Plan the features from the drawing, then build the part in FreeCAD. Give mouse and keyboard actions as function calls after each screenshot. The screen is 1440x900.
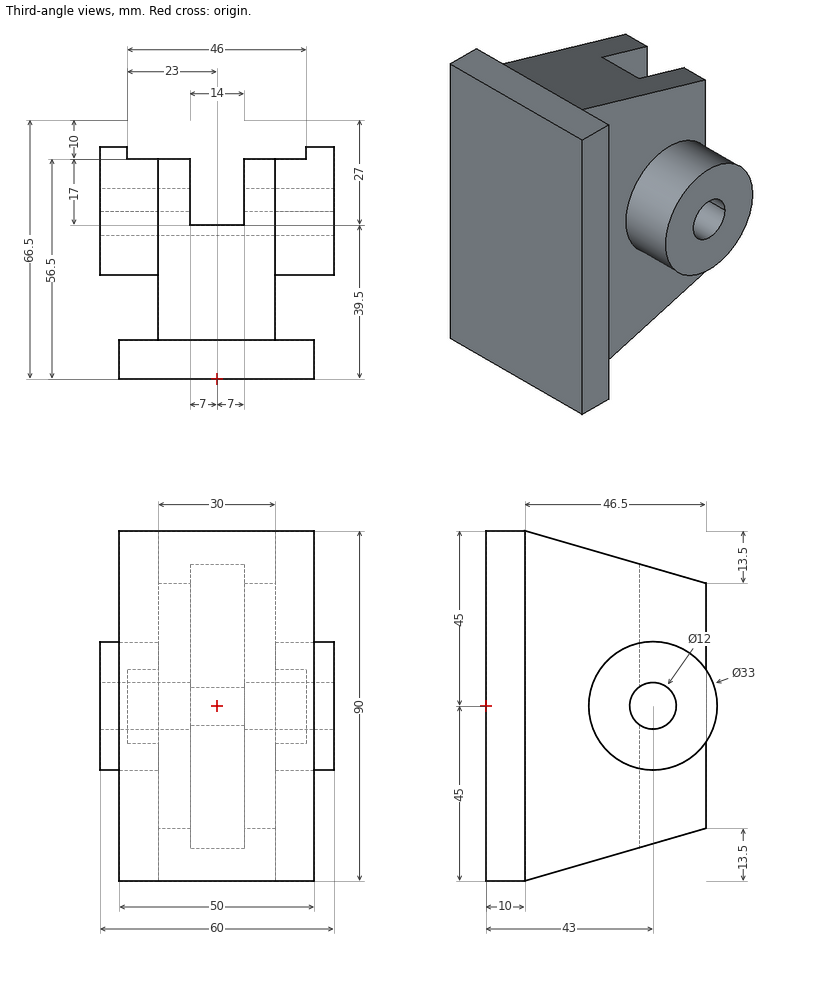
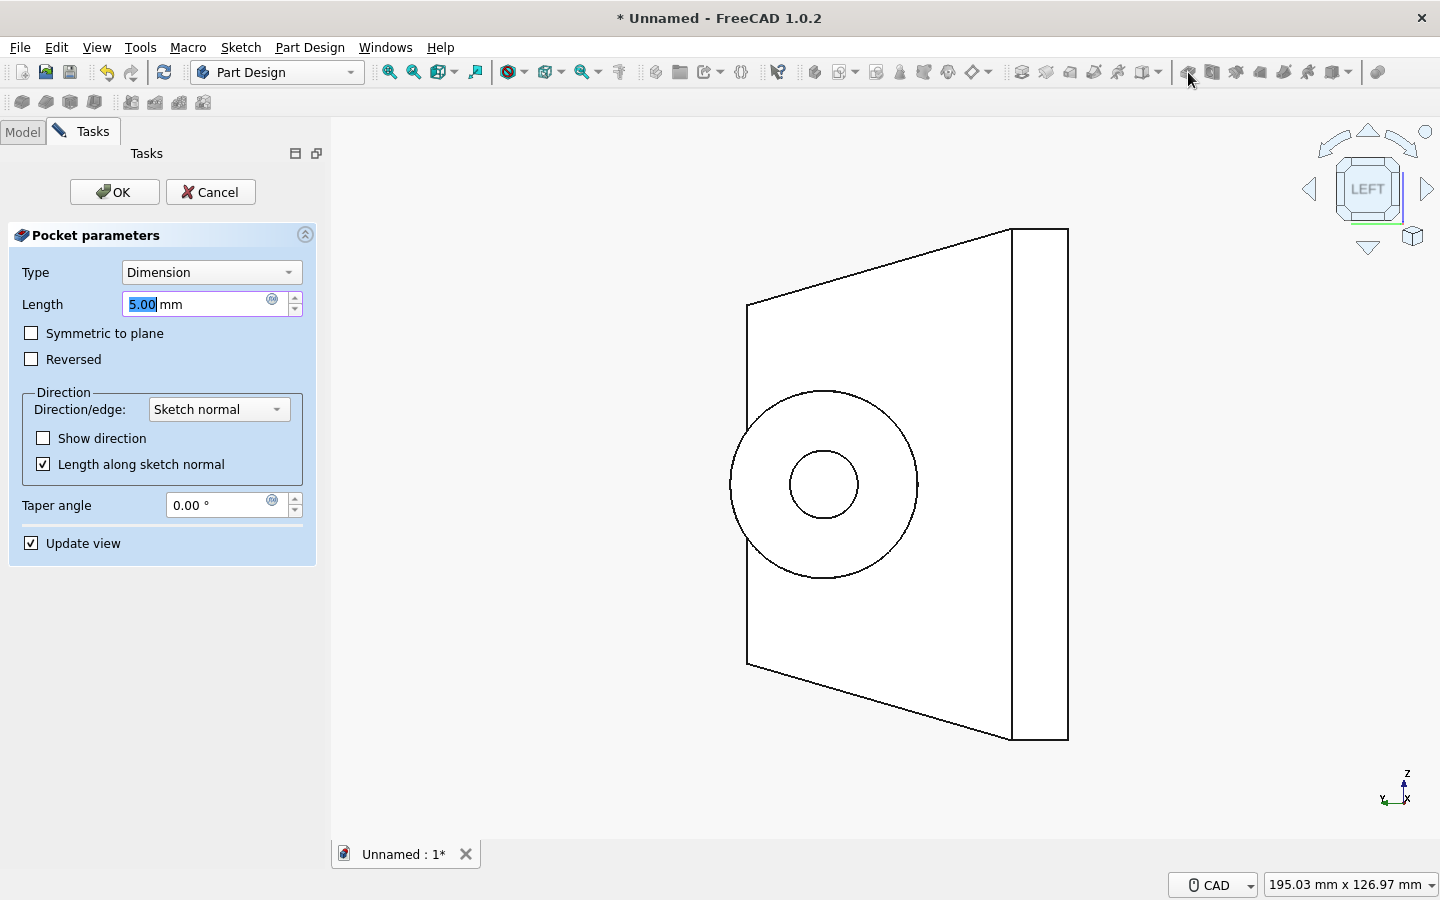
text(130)
key(Tab)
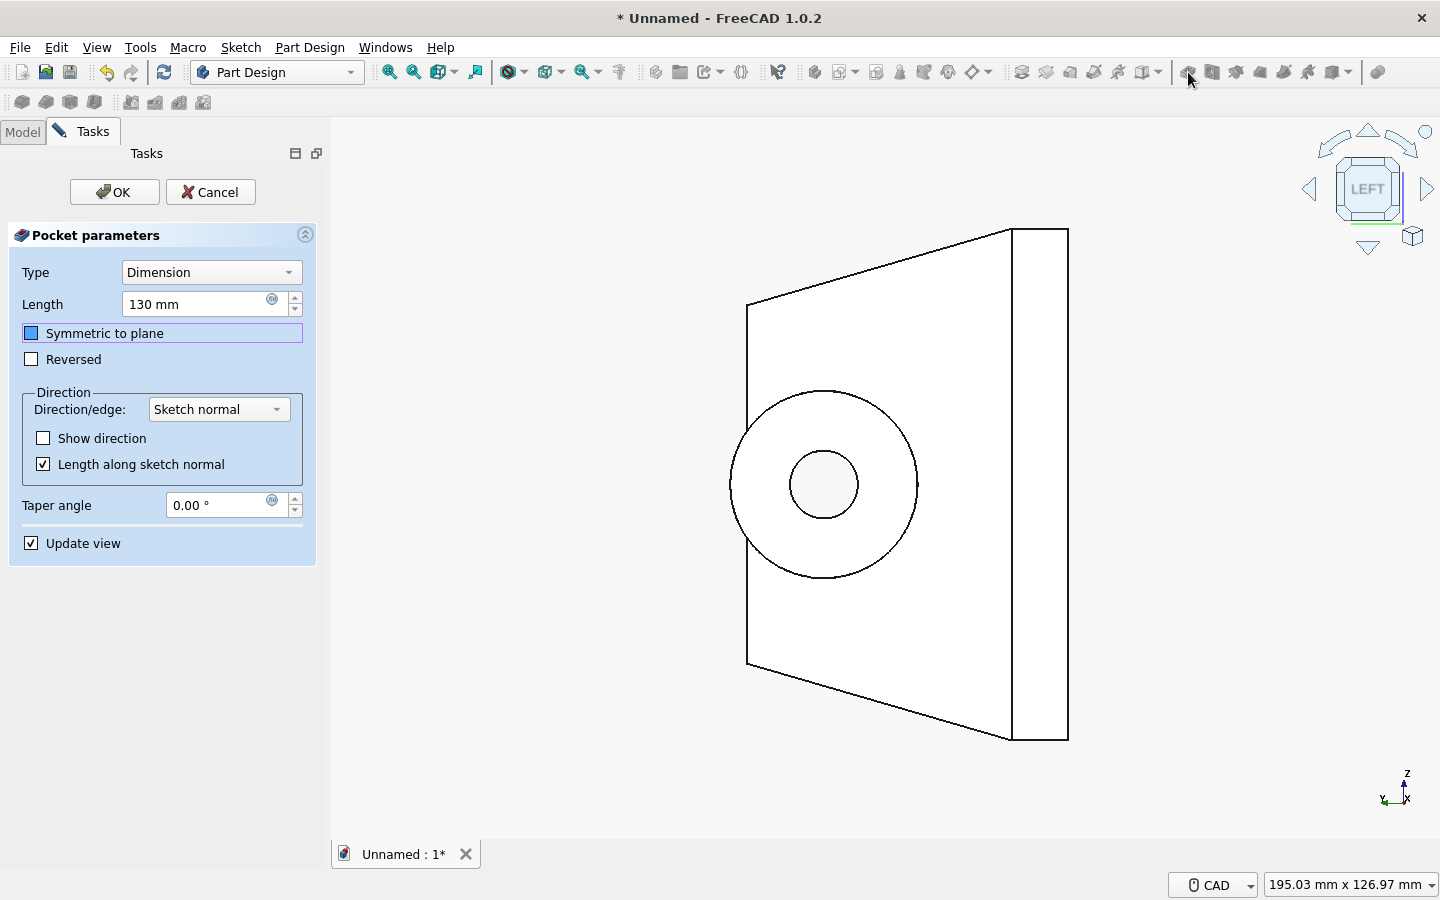
click(30, 333)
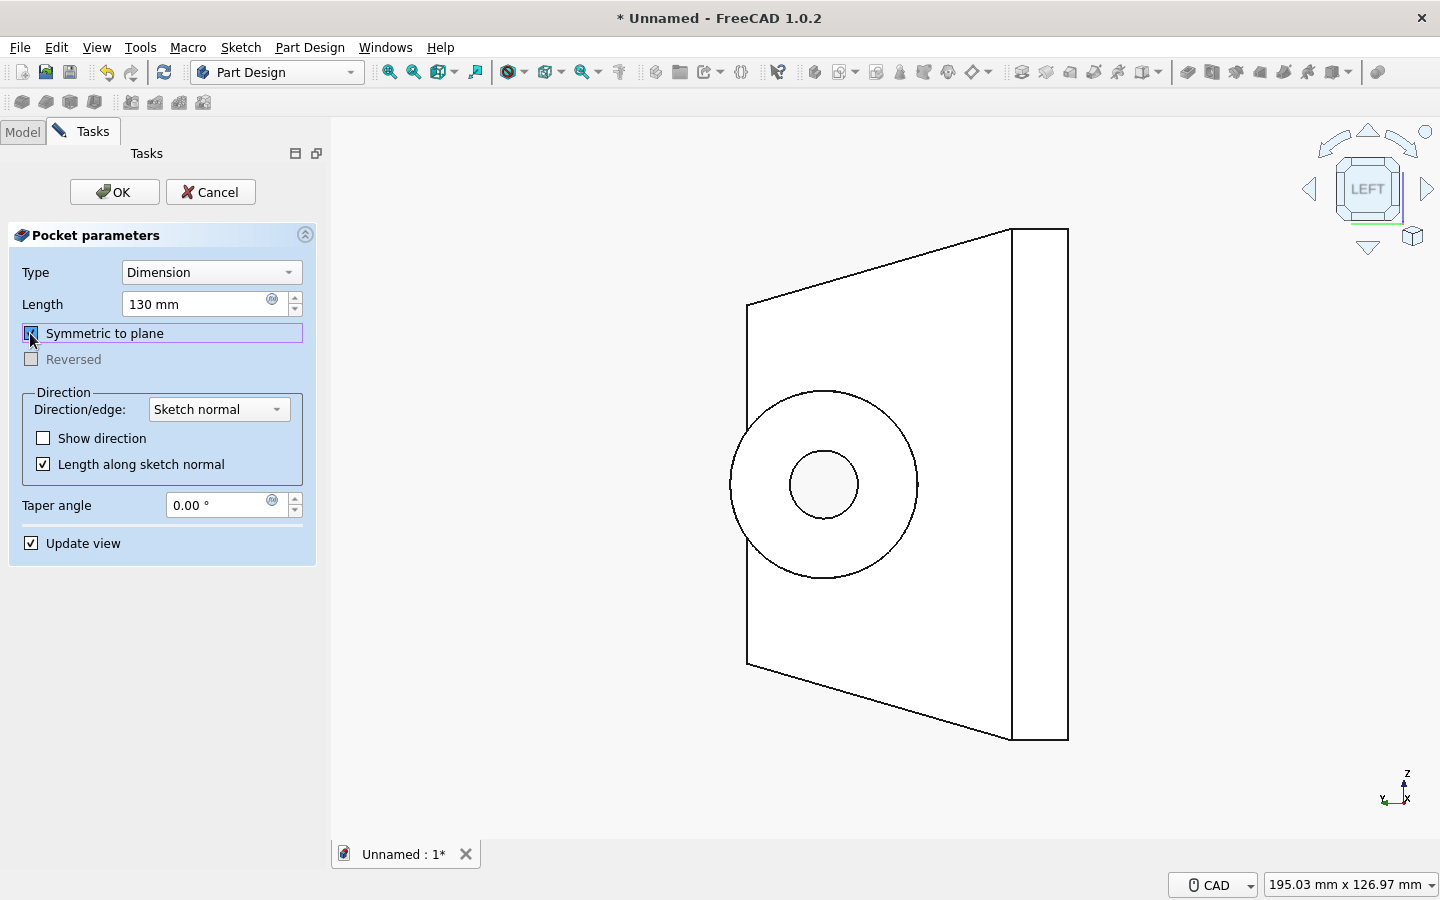
click(115, 192)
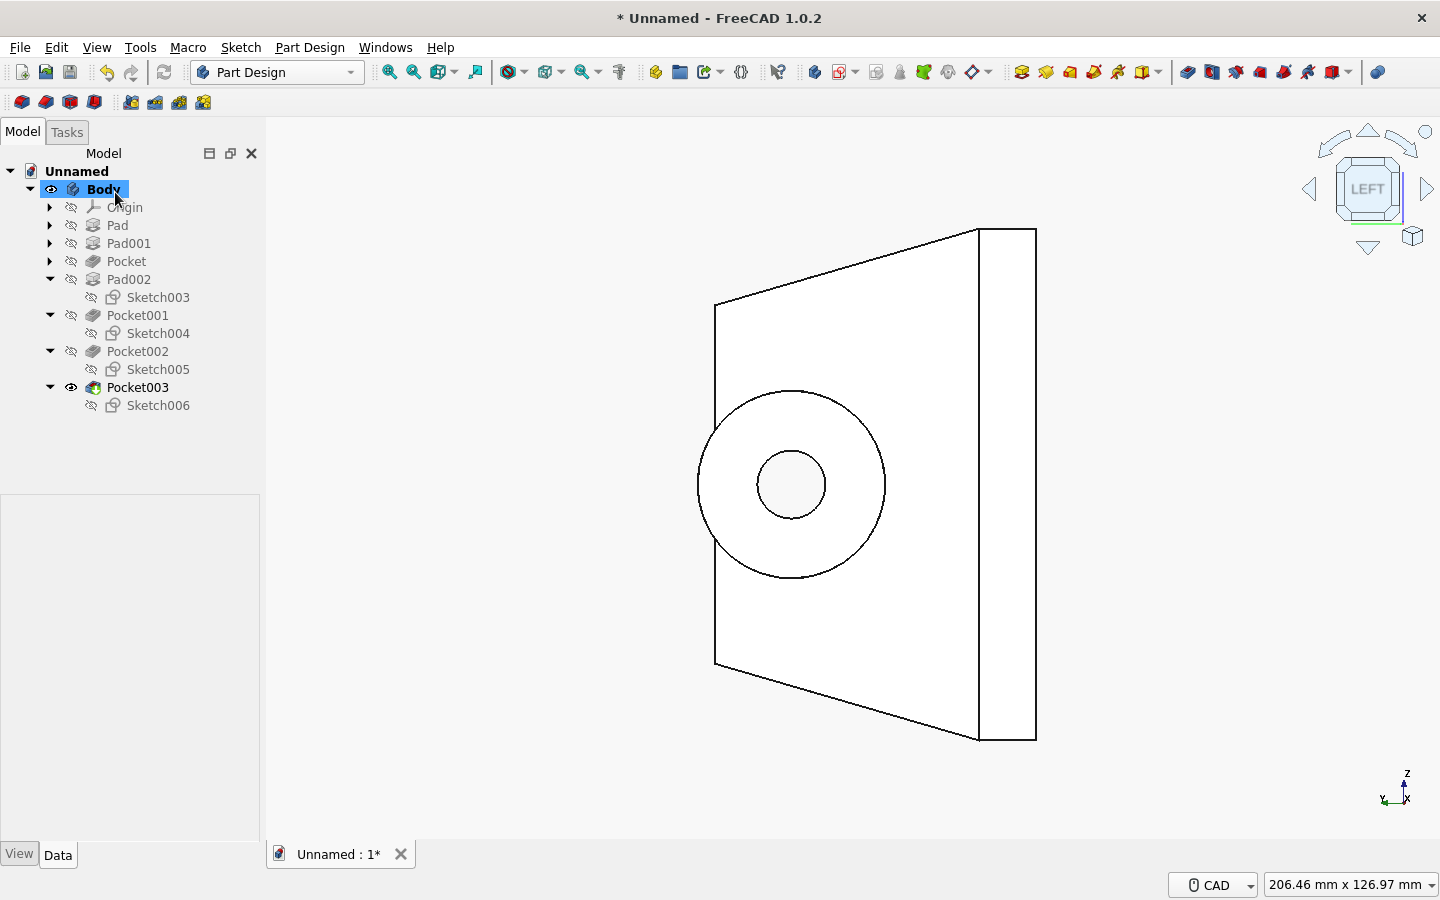
click(840, 72)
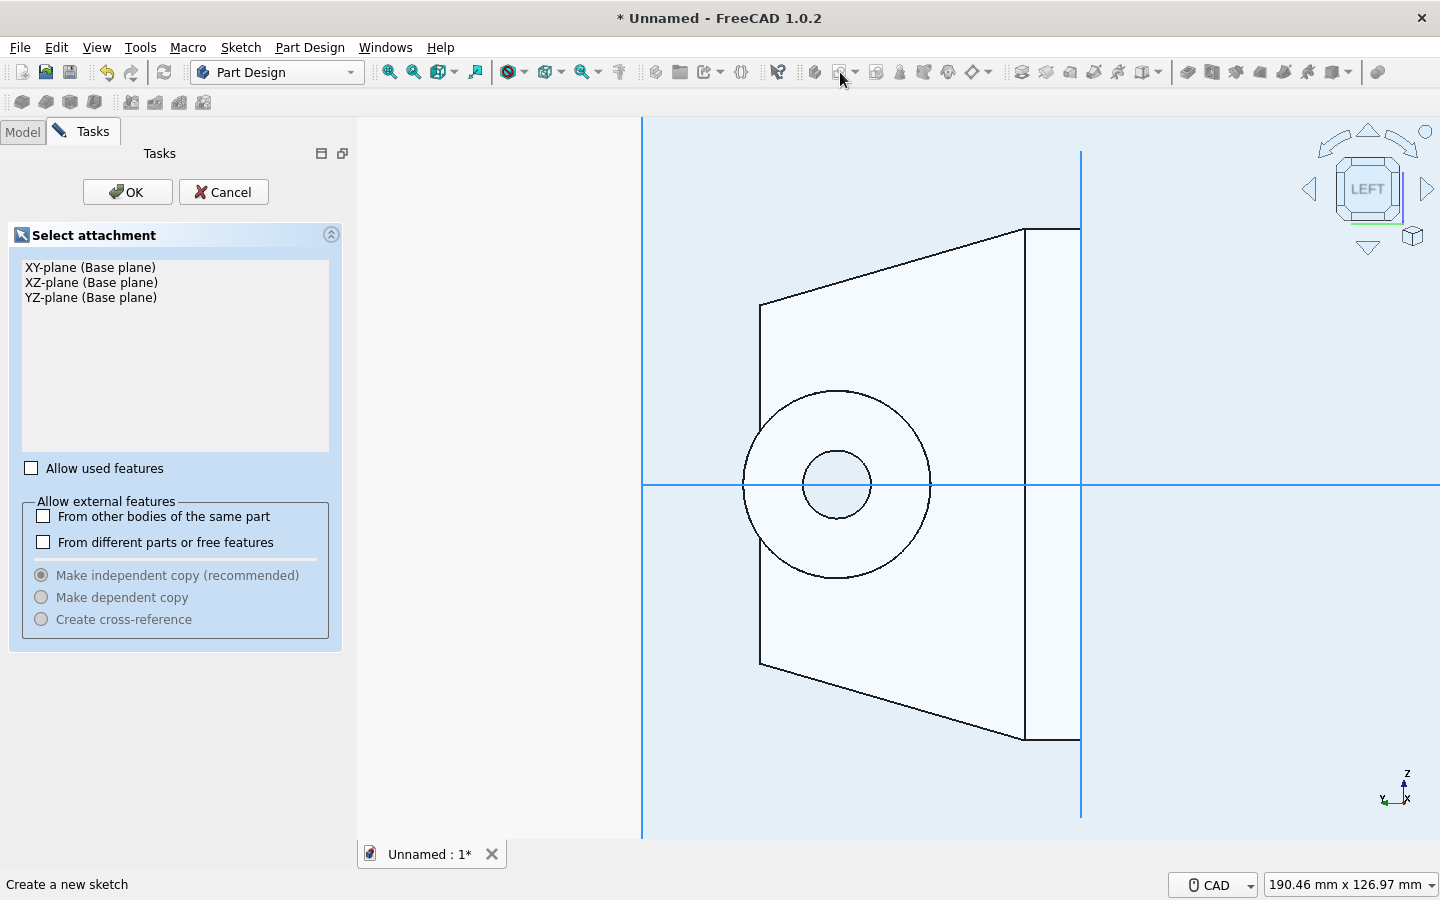
click(82, 268)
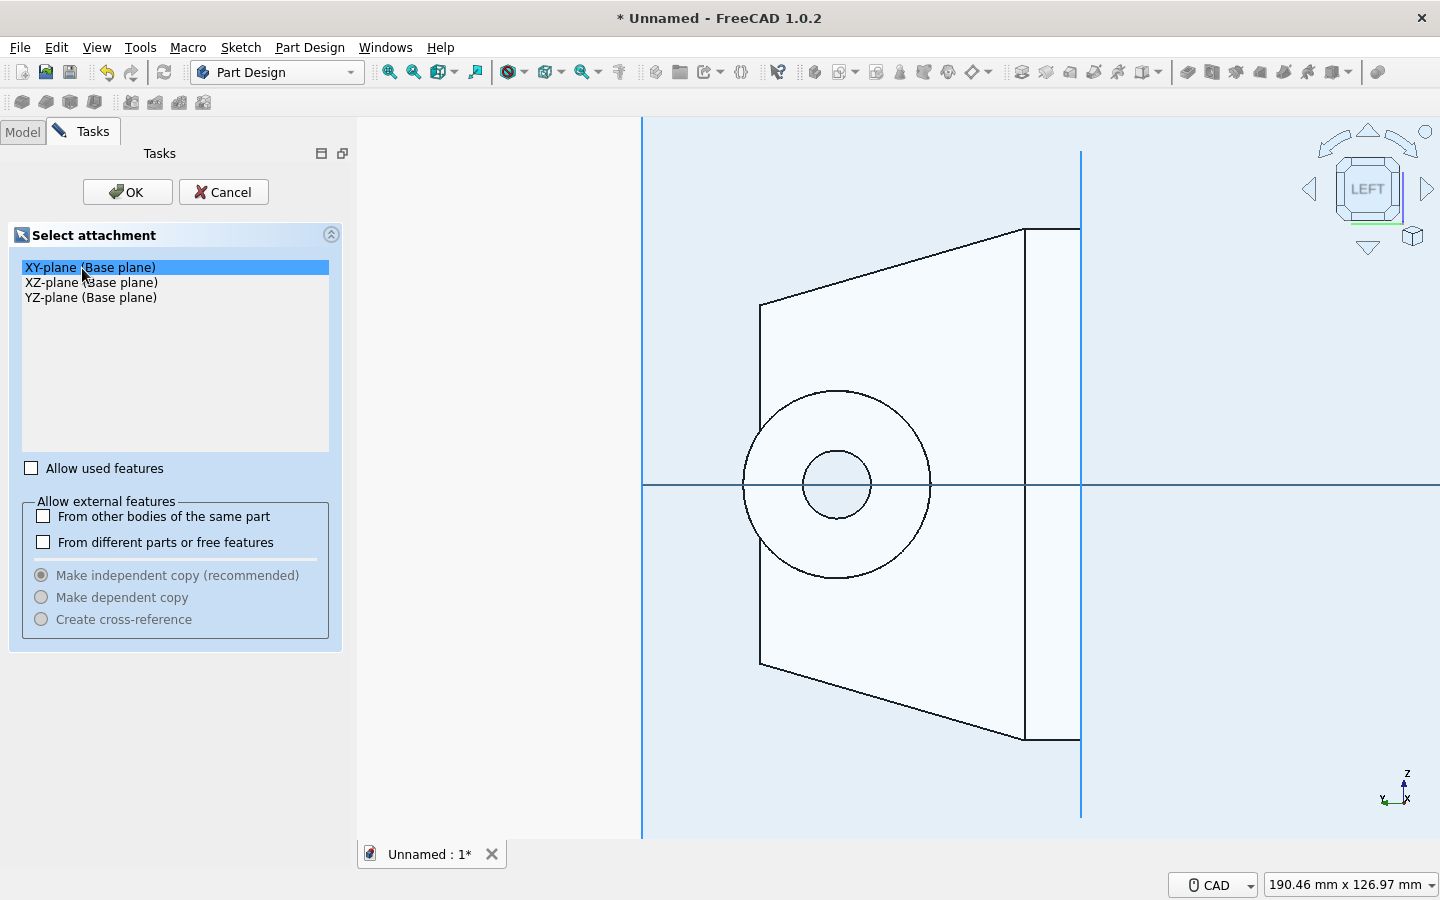
click(128, 192)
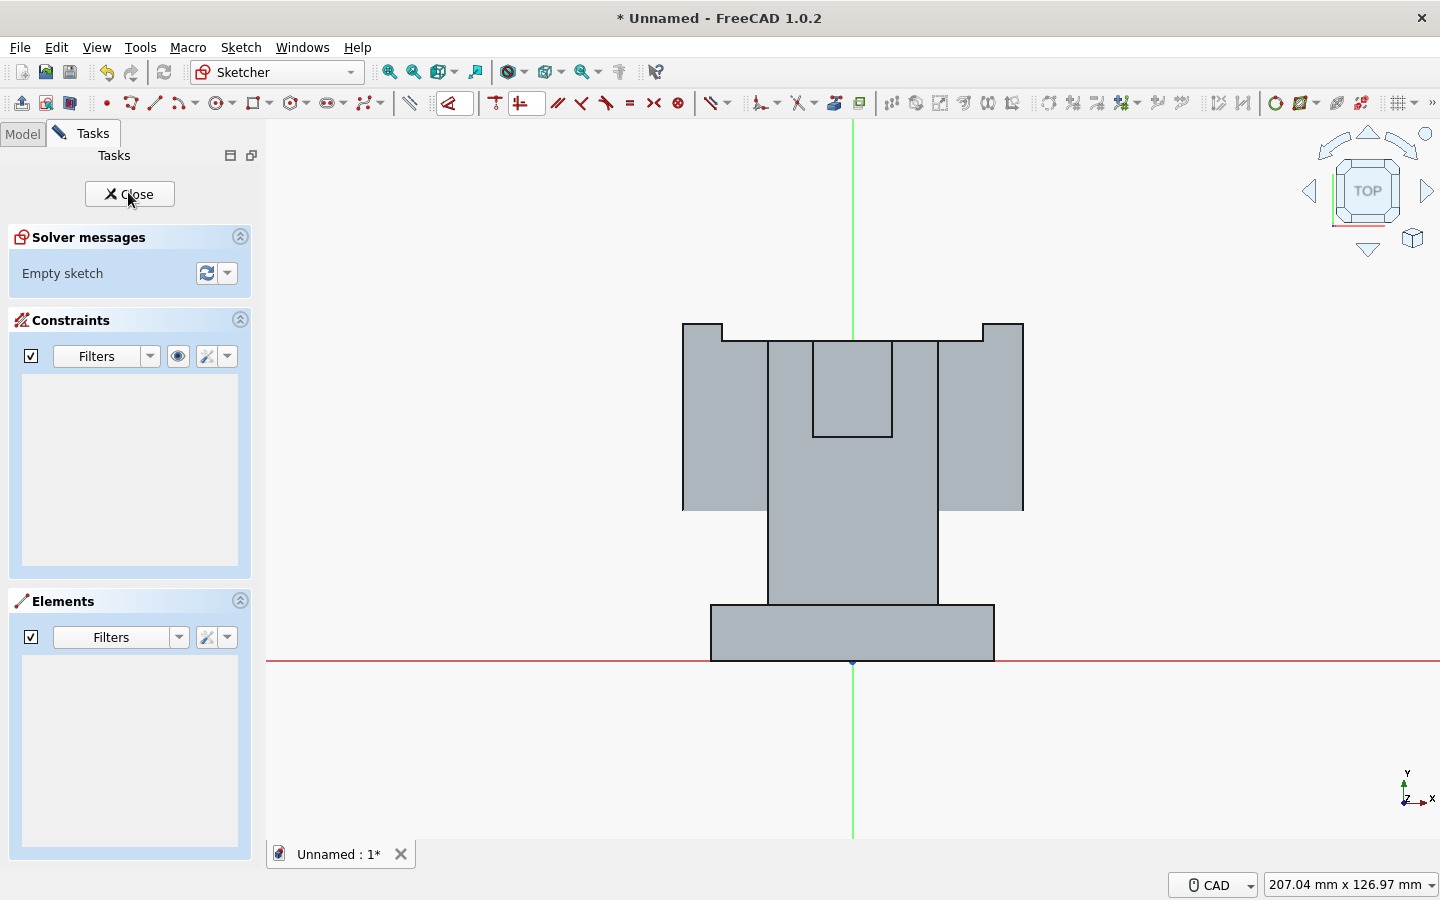
click(70, 104)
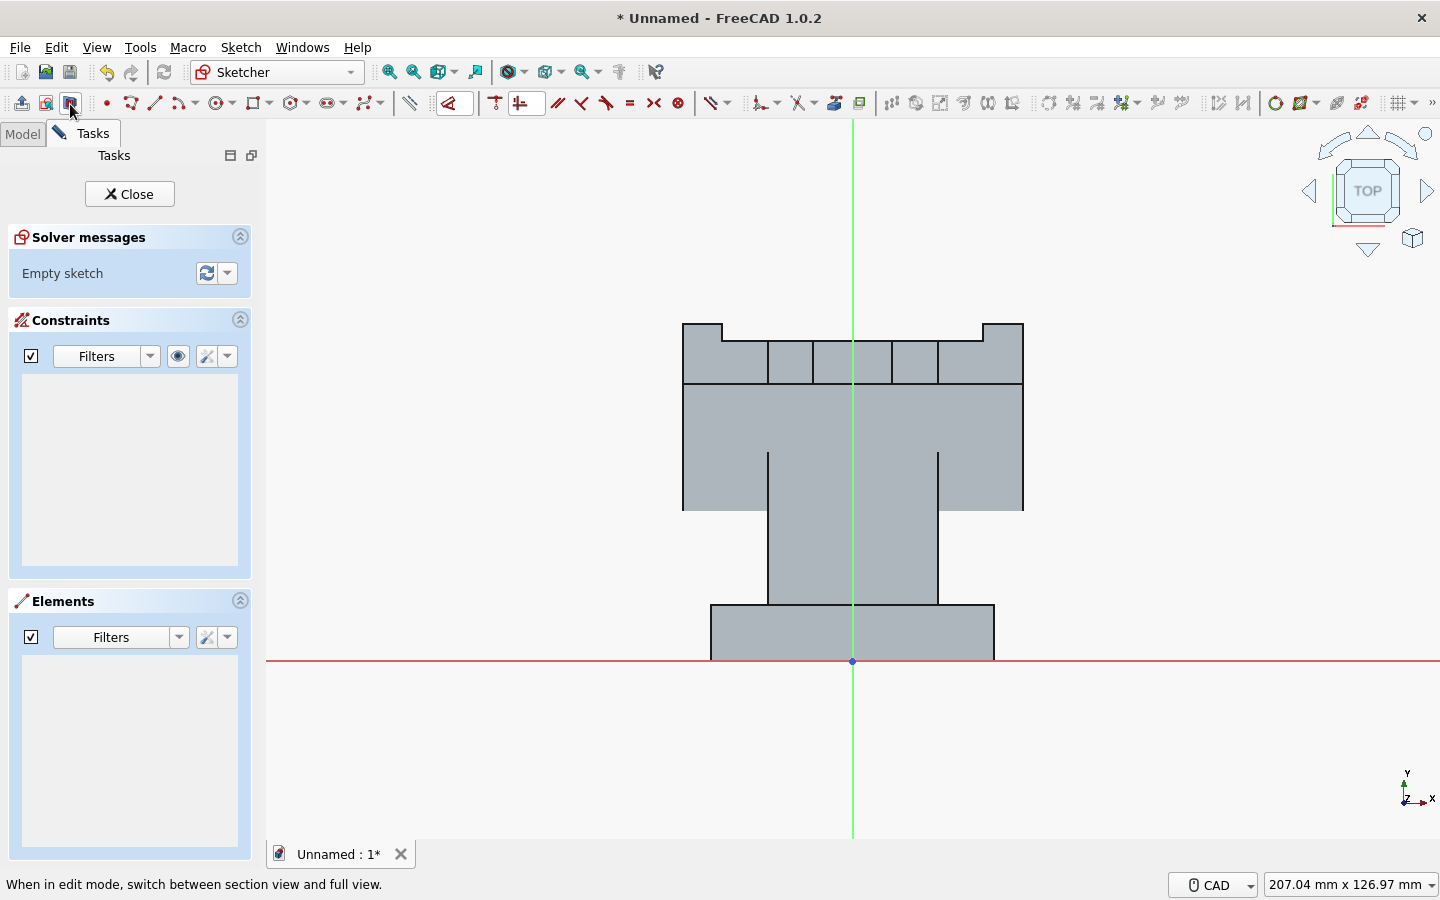
scroll(870, 367, up, 8)